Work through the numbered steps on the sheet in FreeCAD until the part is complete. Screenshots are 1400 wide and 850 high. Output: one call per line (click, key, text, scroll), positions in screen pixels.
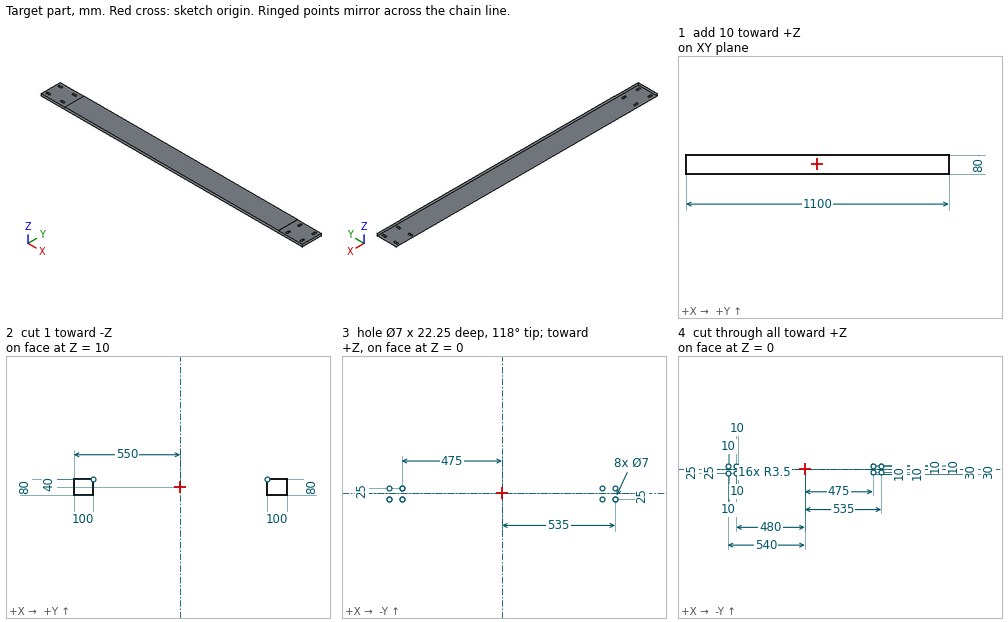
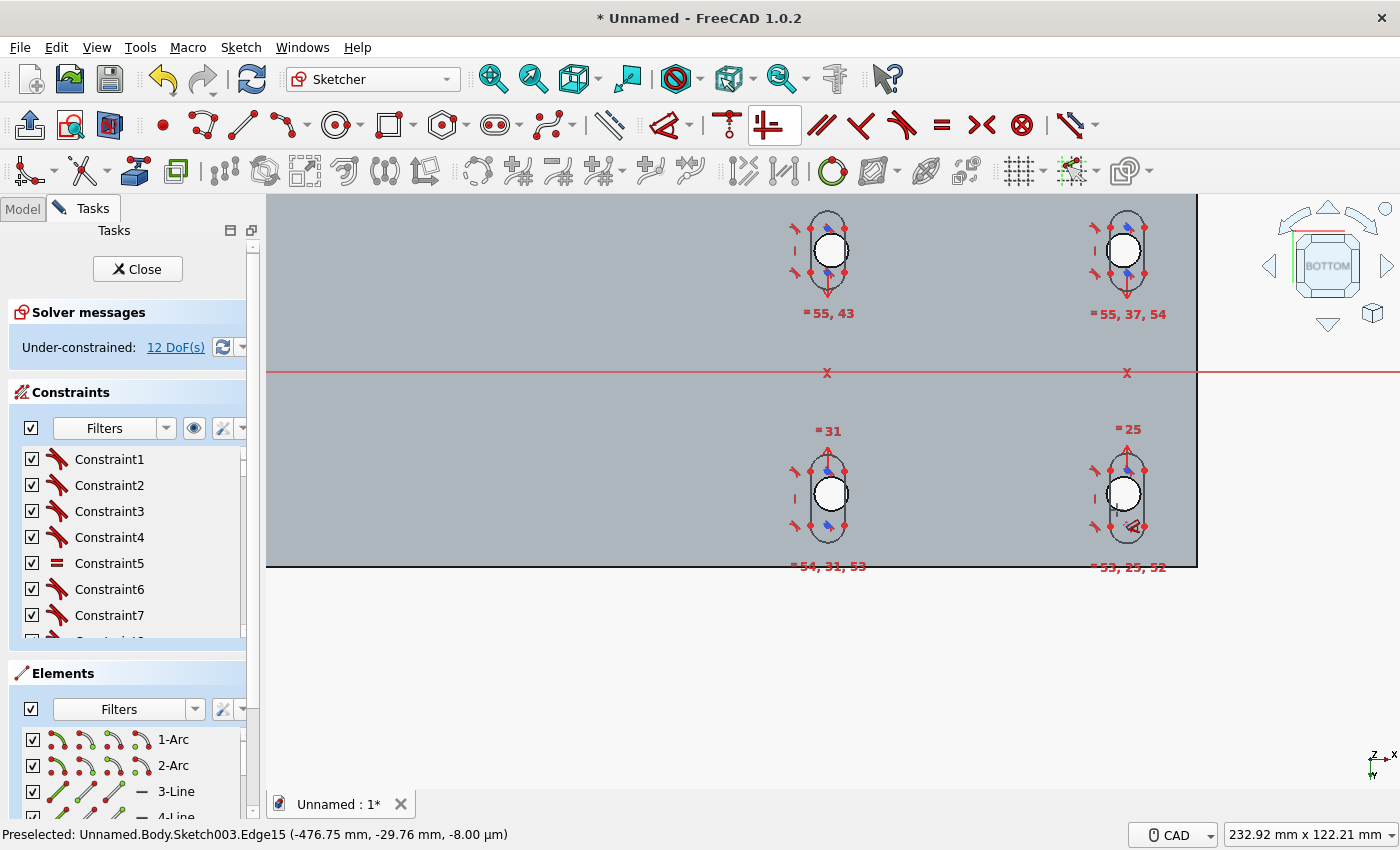
click(1110, 510)
click(1076, 498)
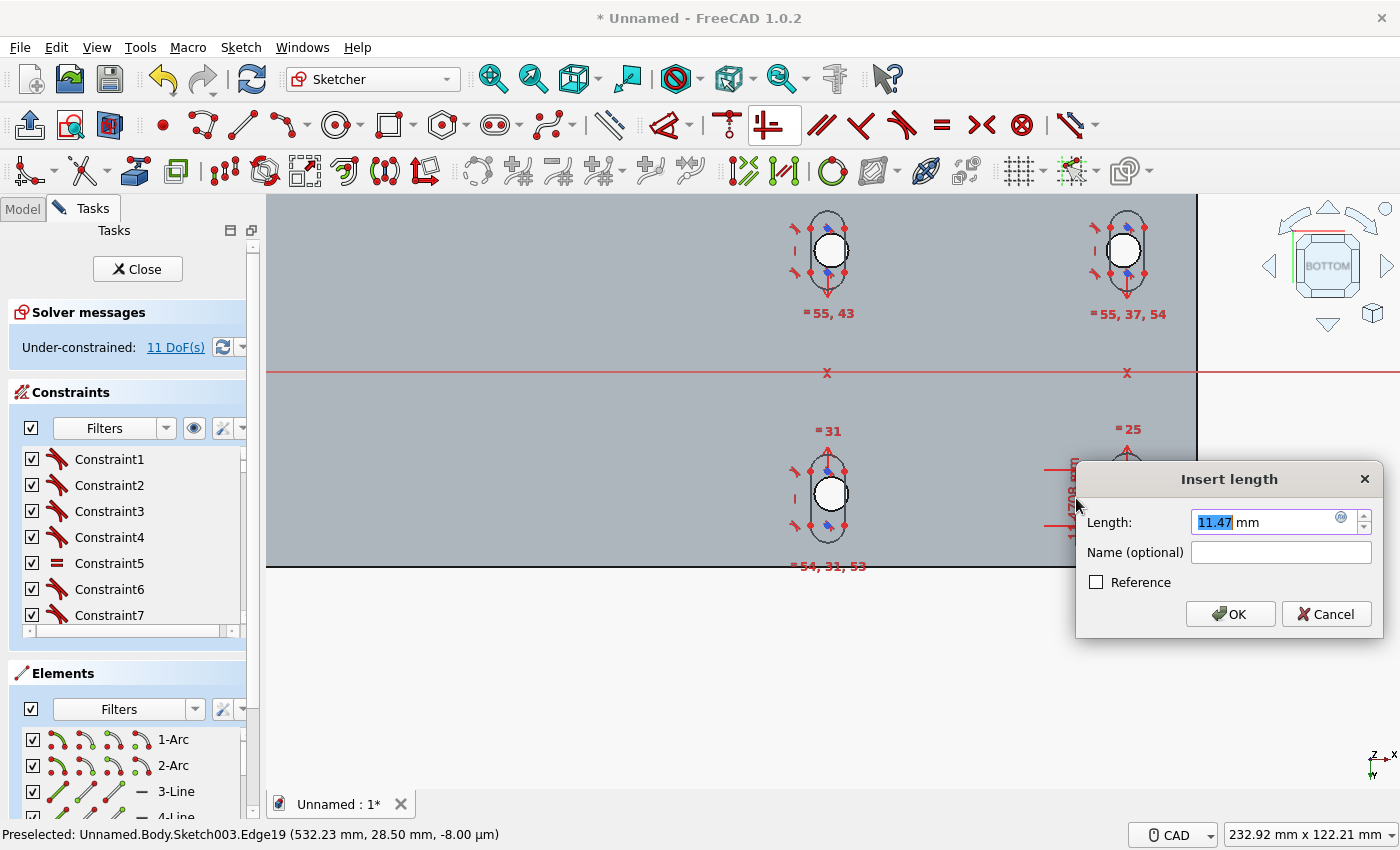
text(10)
key(Return)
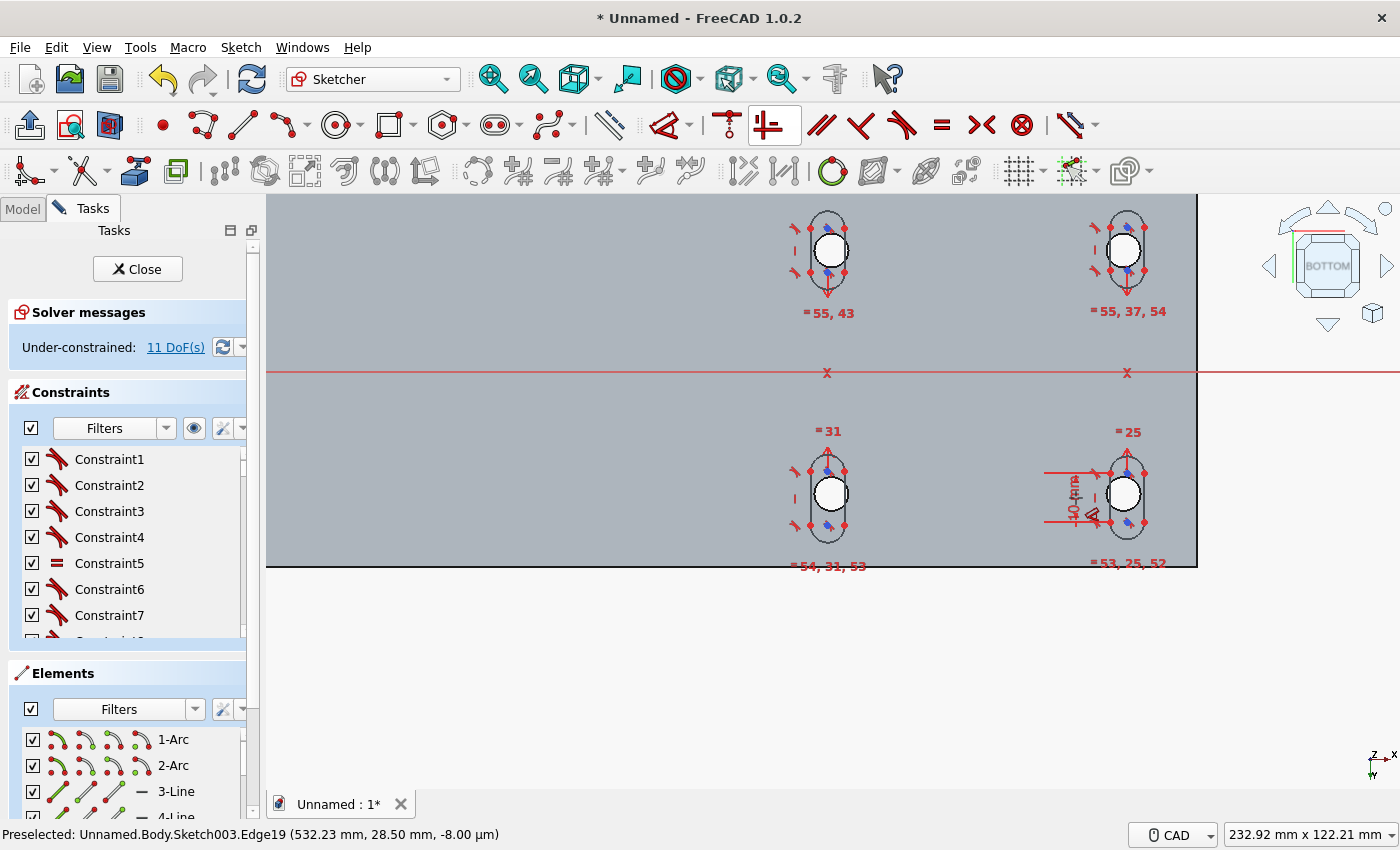
click(811, 509)
click(777, 499)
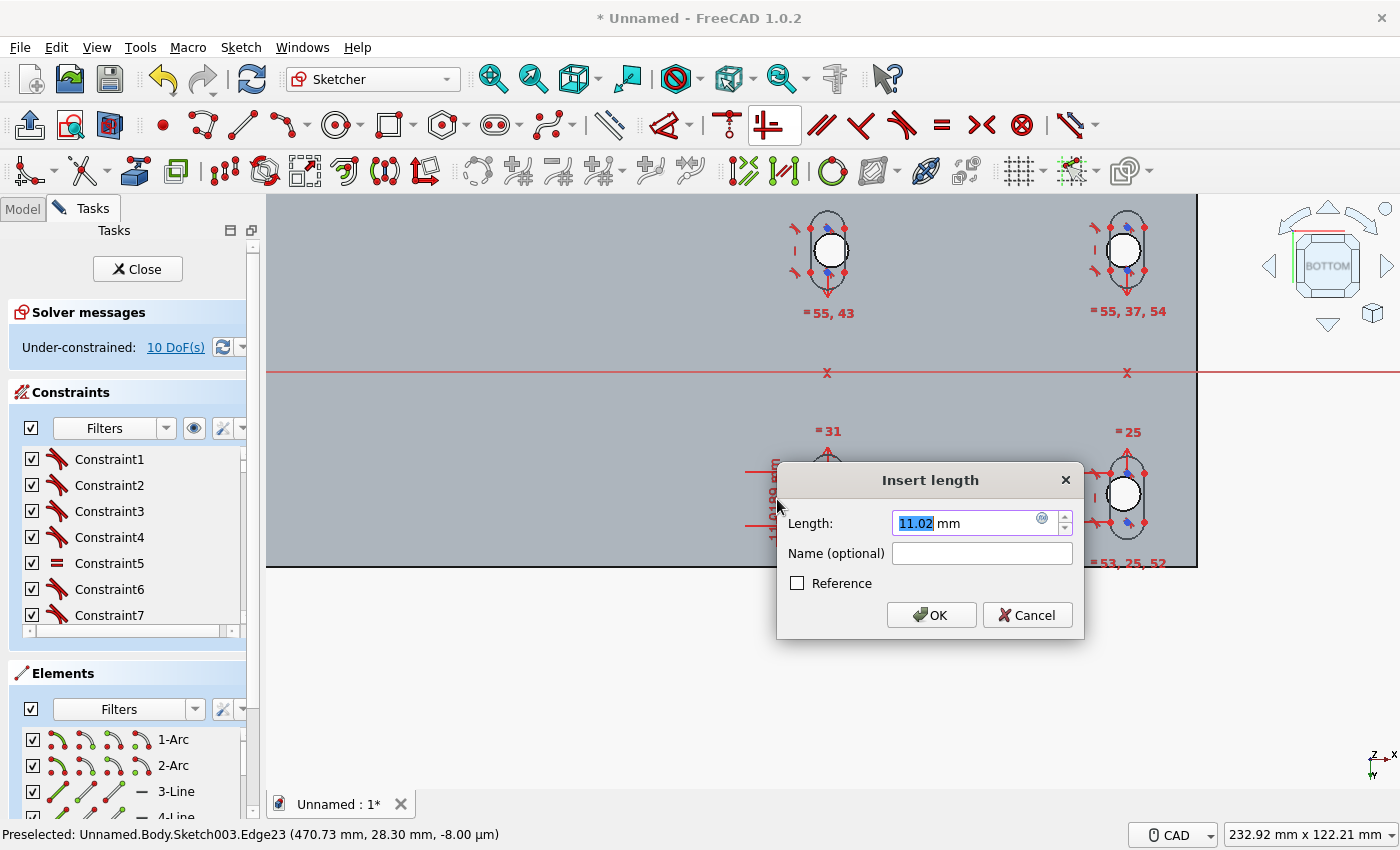
text(10)
key(Return)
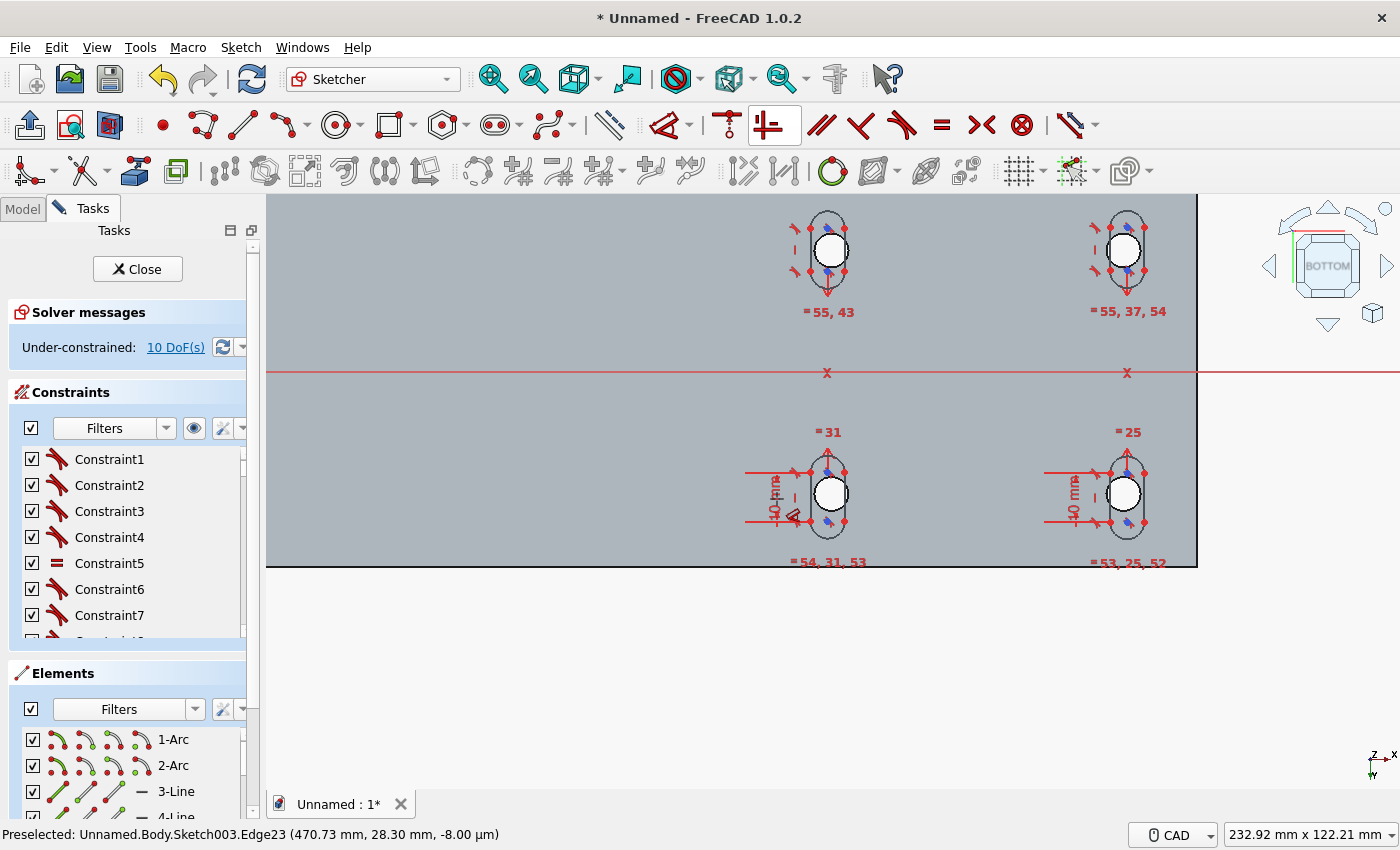
click(1110, 258)
click(1076, 249)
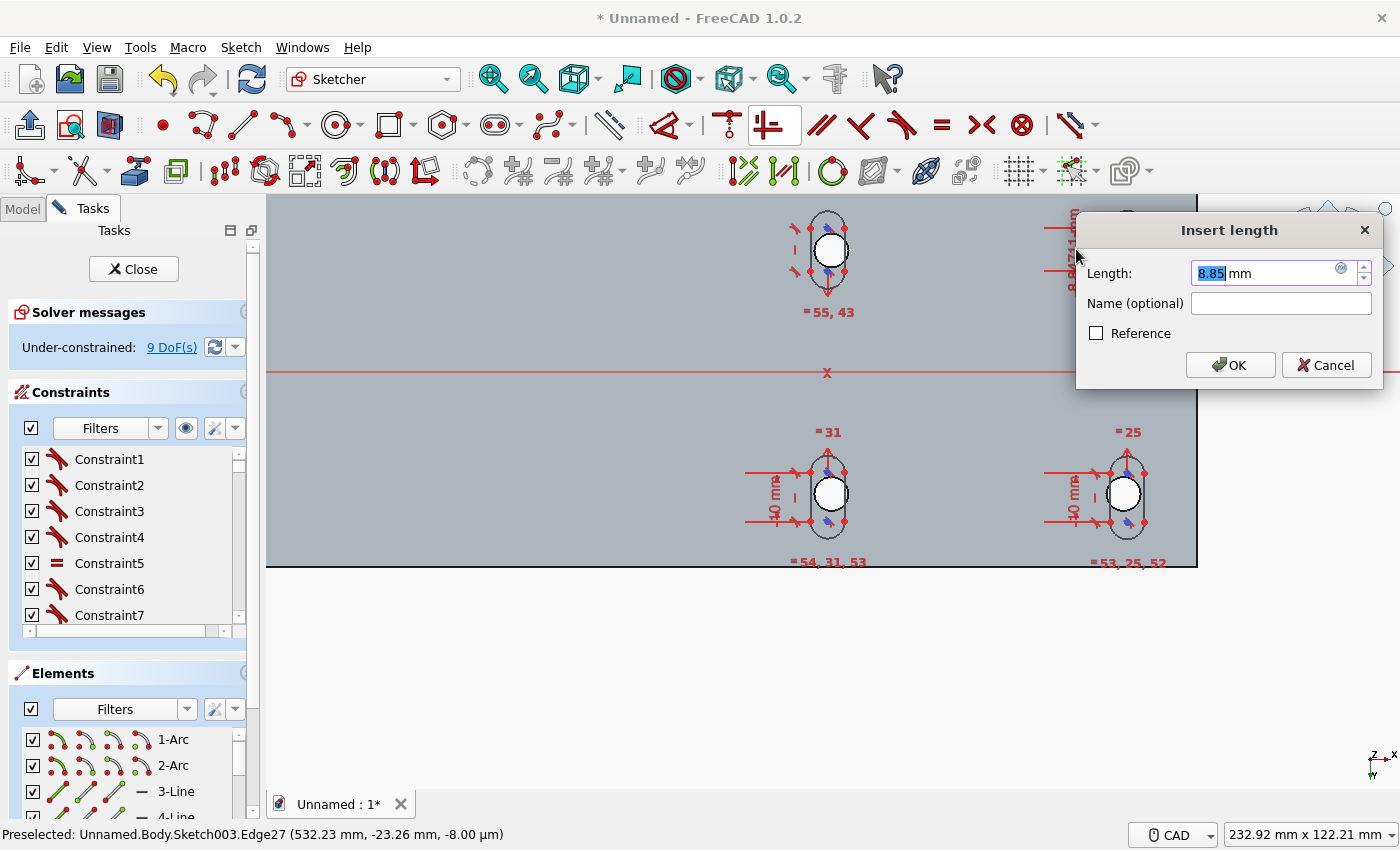
text(10)
key(Return)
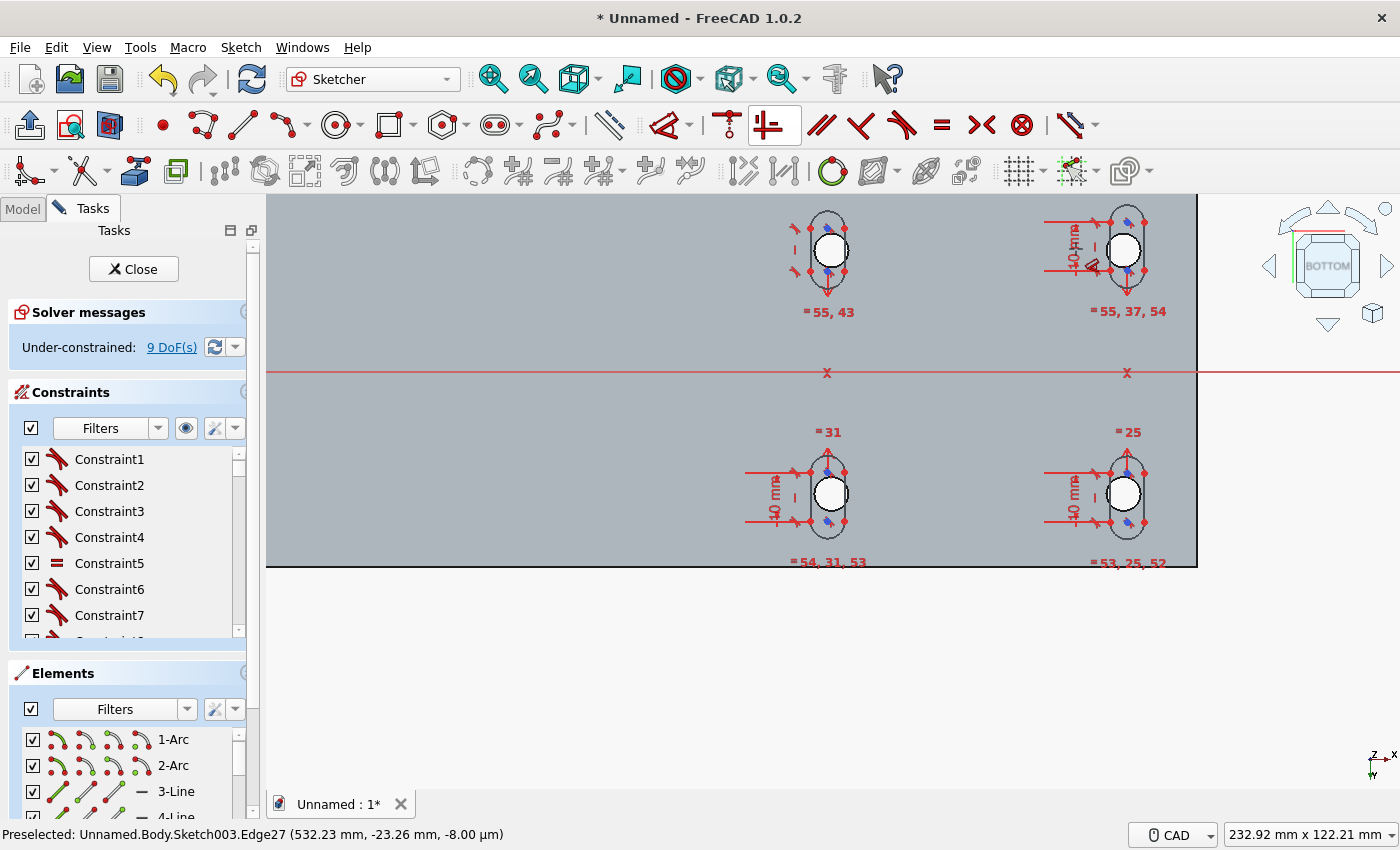
click(811, 259)
click(777, 250)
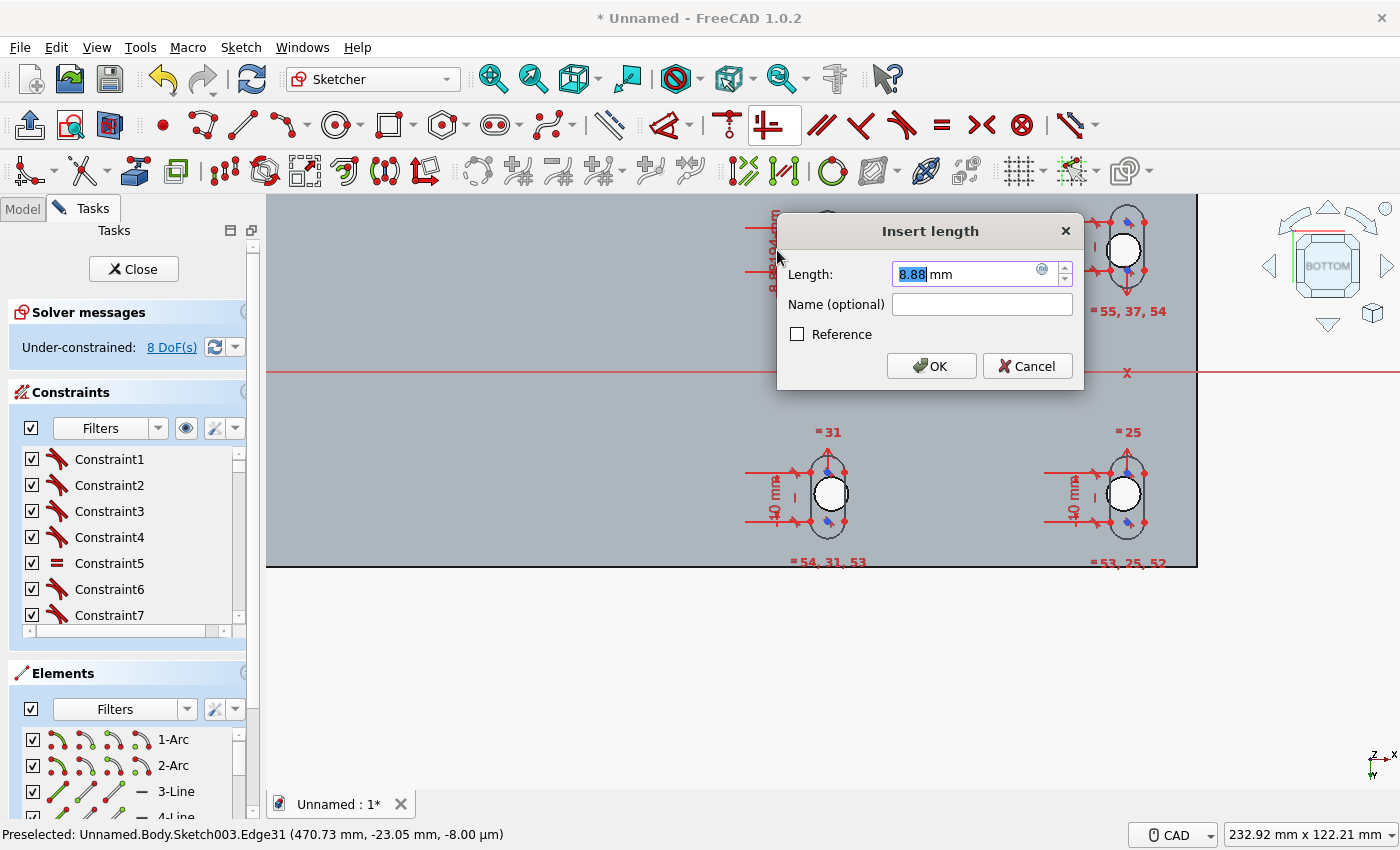
text(10)
key(Return)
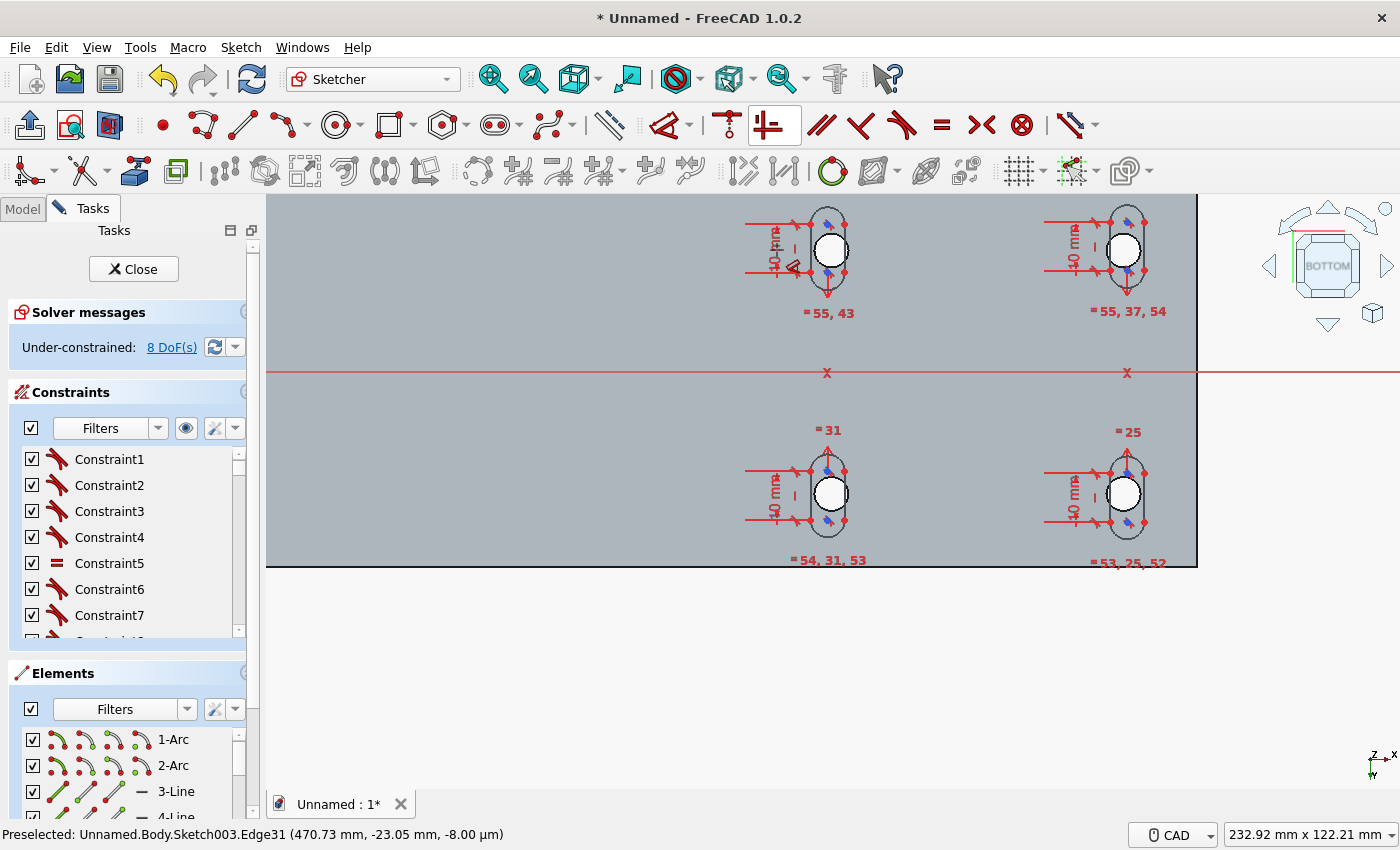
click(1110, 522)
click(1144, 447)